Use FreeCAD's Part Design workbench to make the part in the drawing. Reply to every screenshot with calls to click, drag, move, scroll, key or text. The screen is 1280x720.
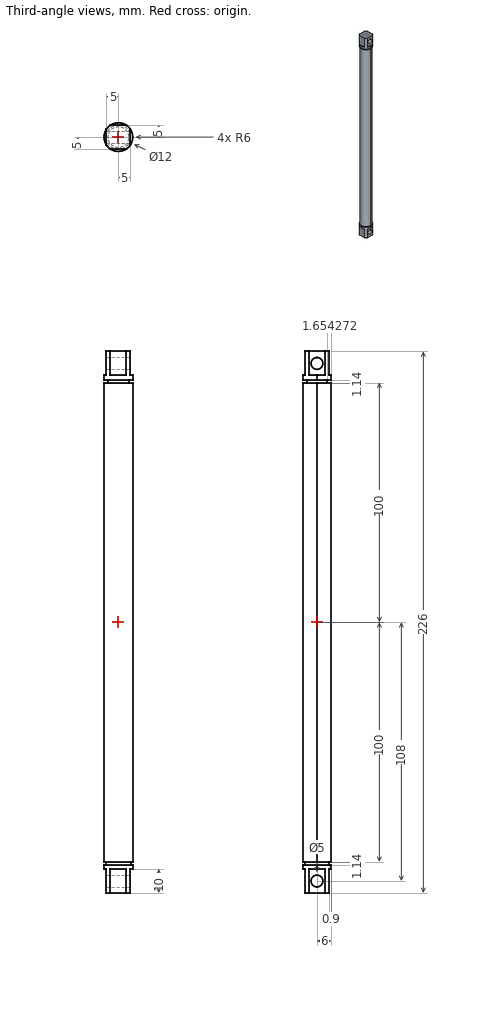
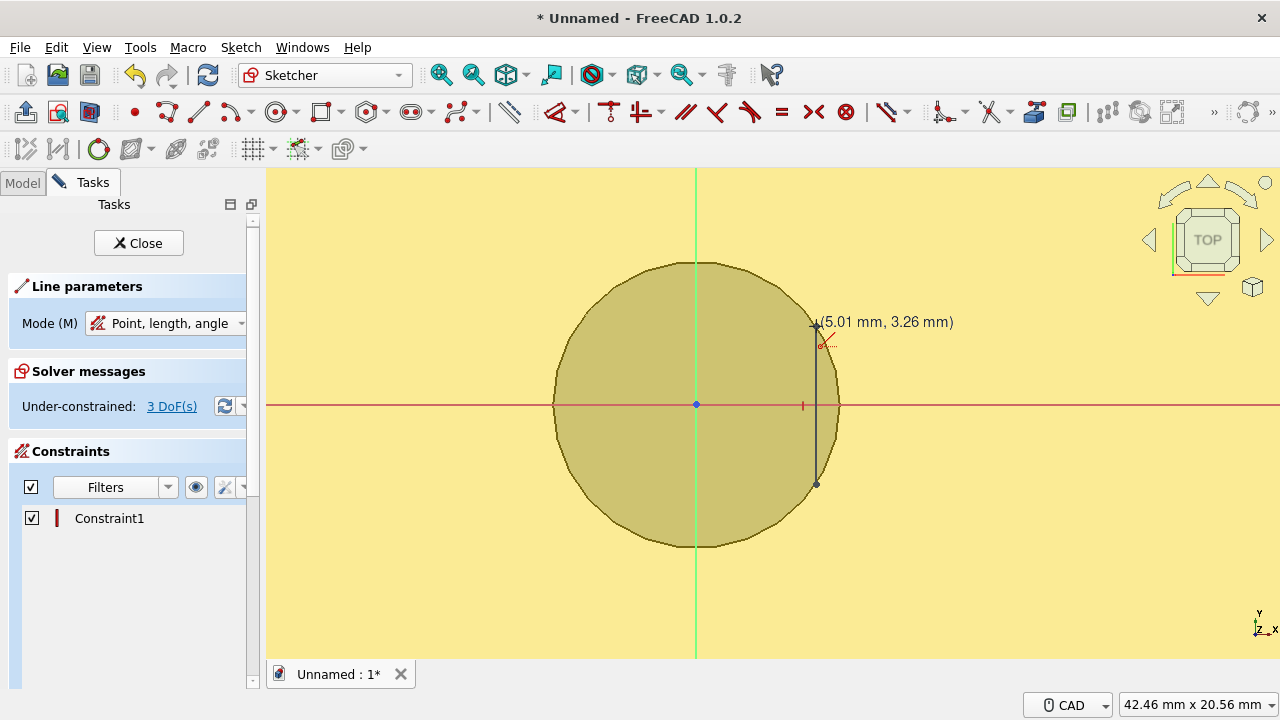
click(254, 112)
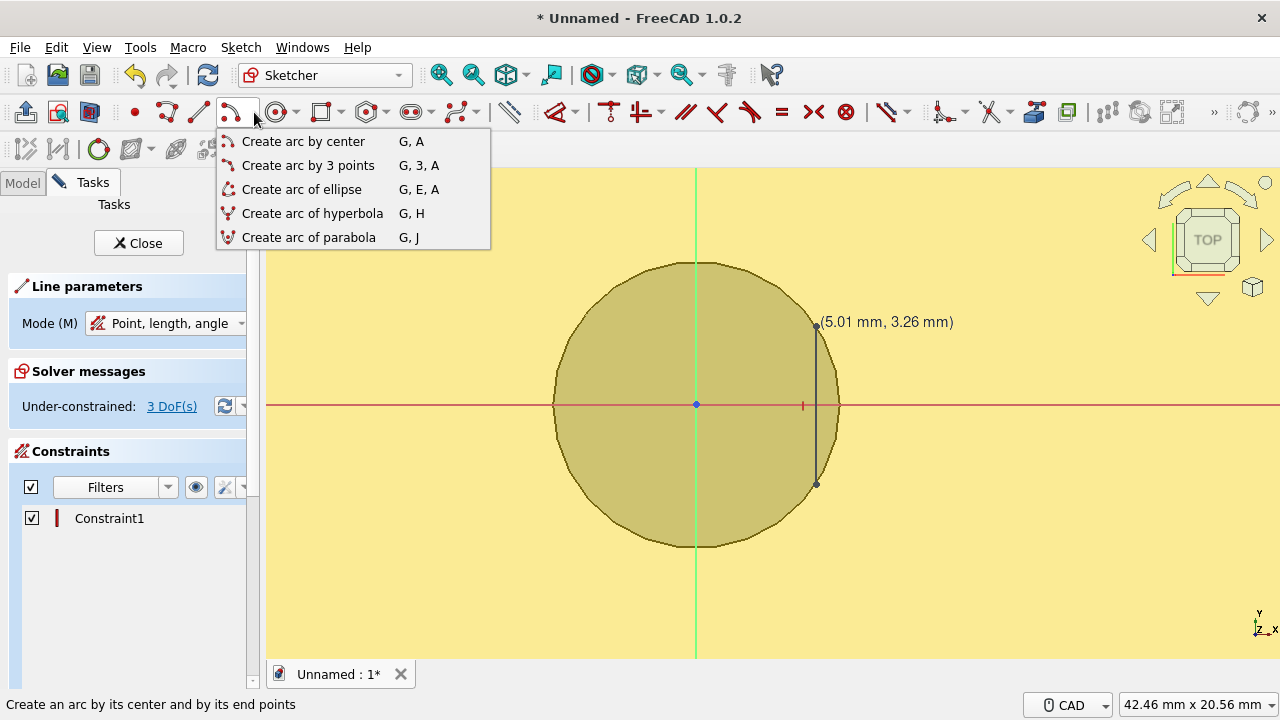
click(354, 165)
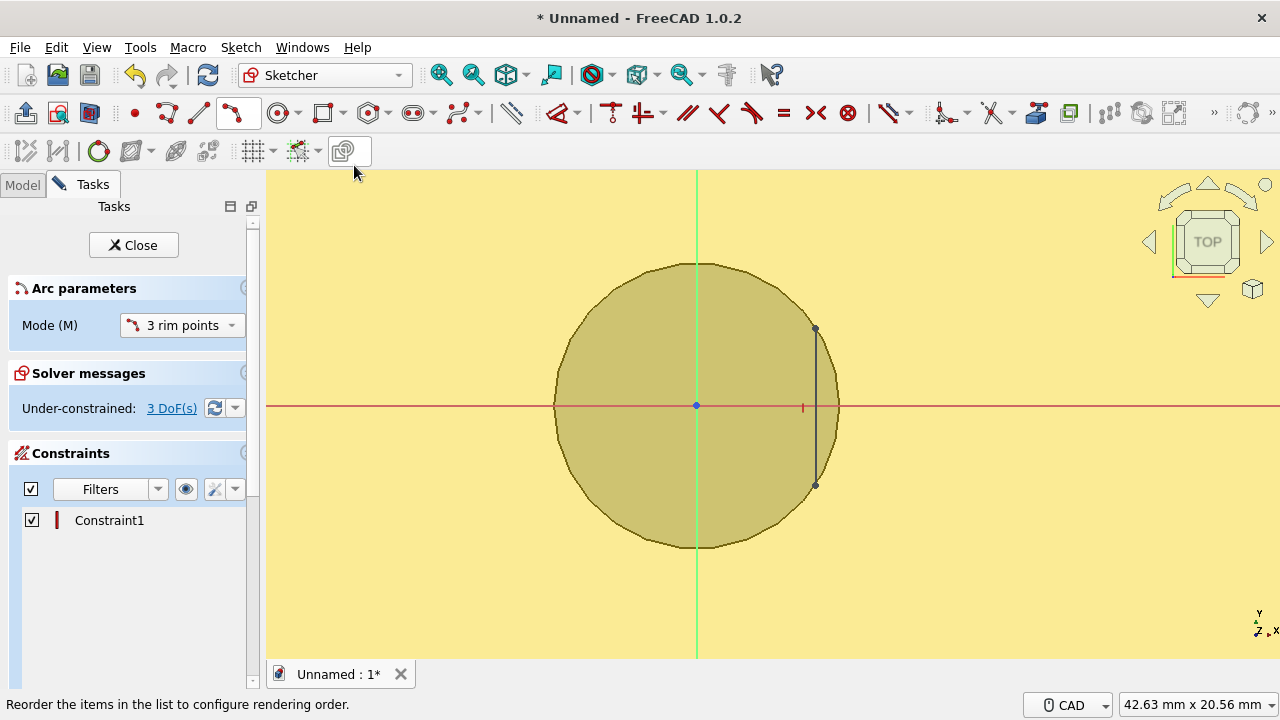
click(816, 328)
click(816, 486)
click(838, 423)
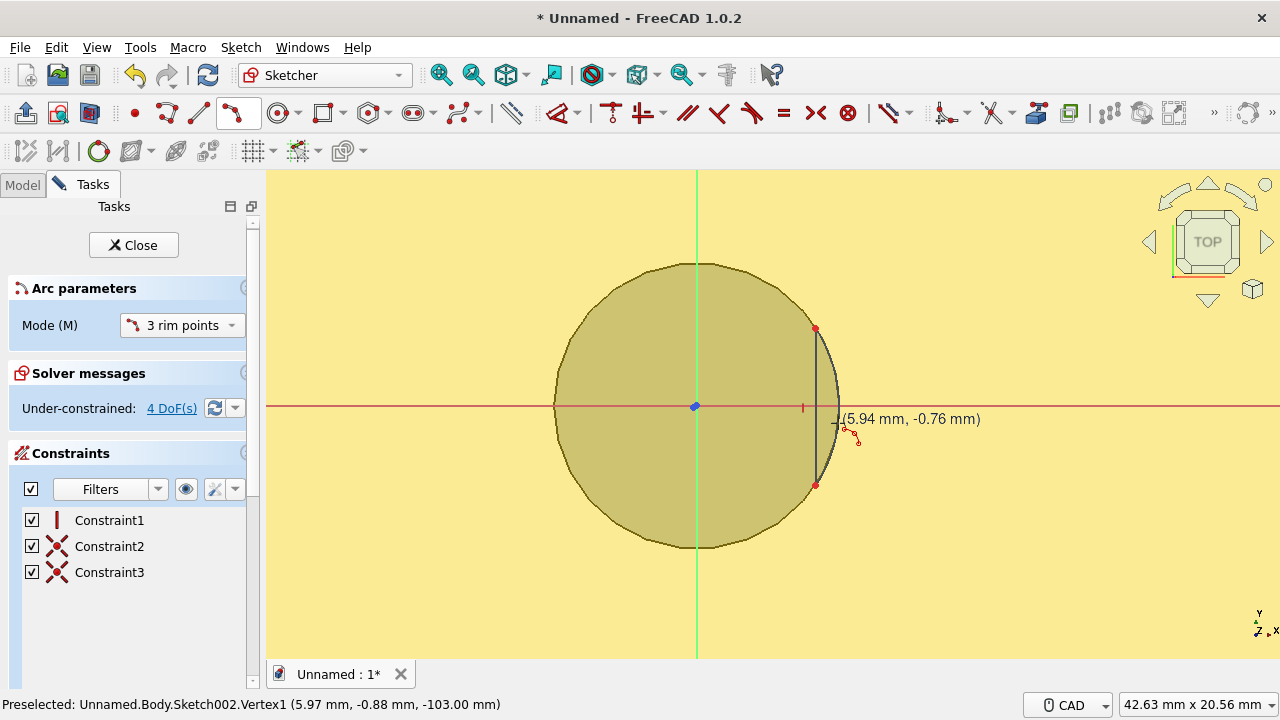
click(200, 114)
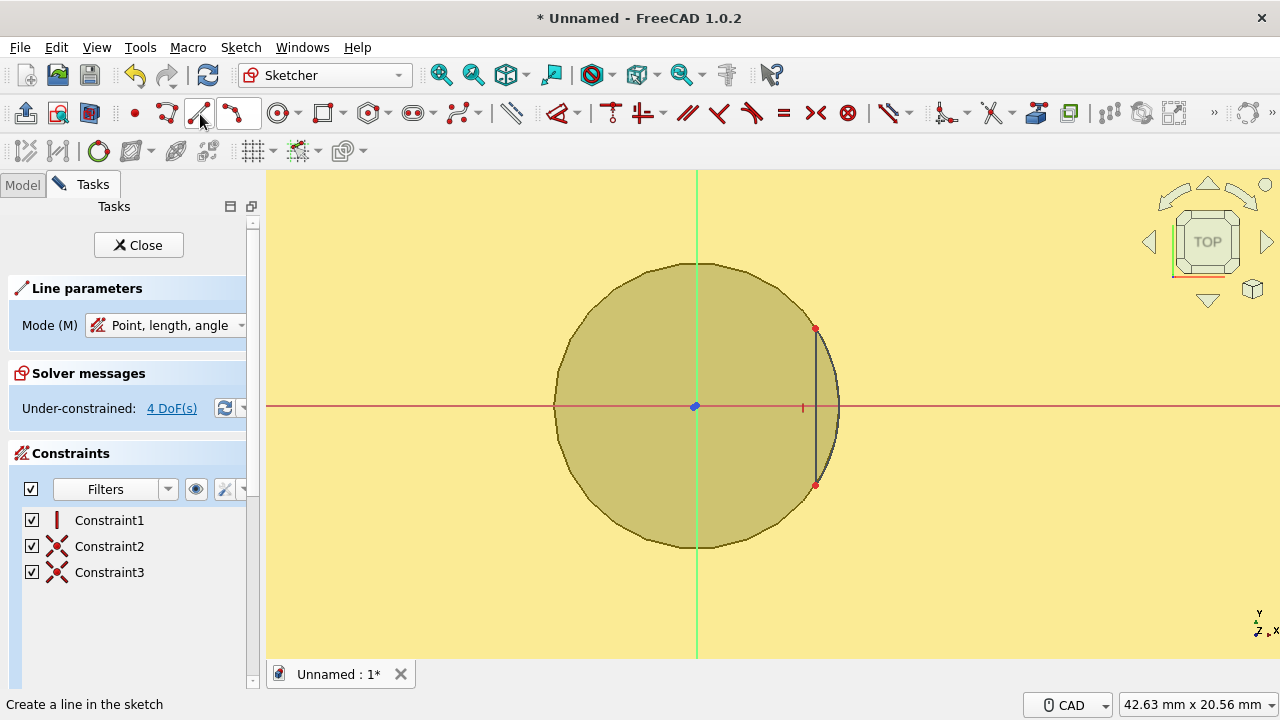
click(578, 327)
click(578, 485)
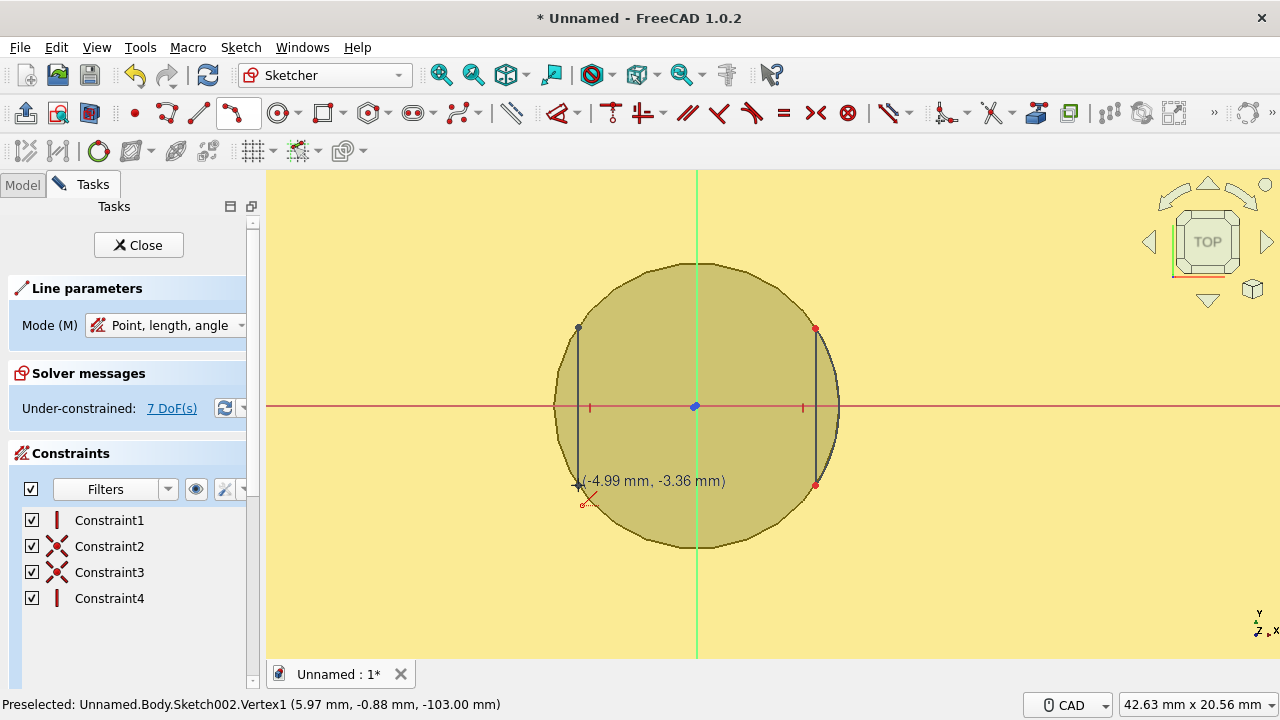
click(232, 114)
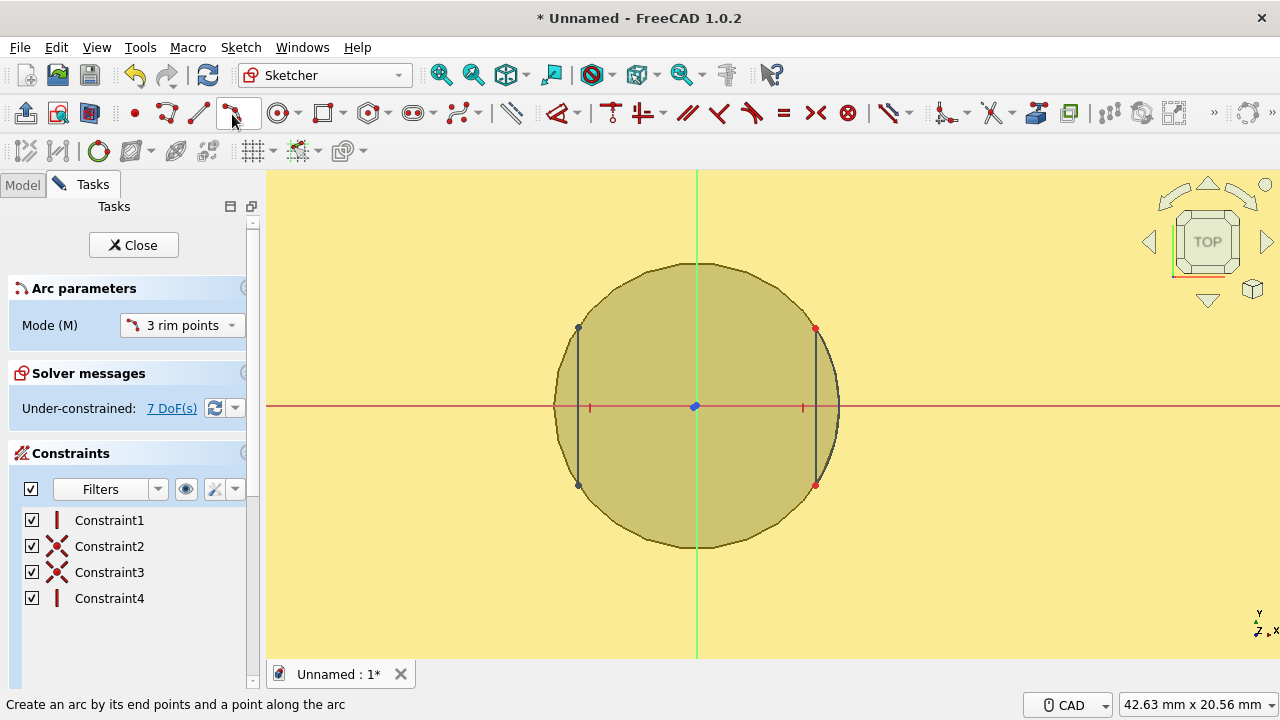
click(578, 486)
click(578, 328)
click(555, 389)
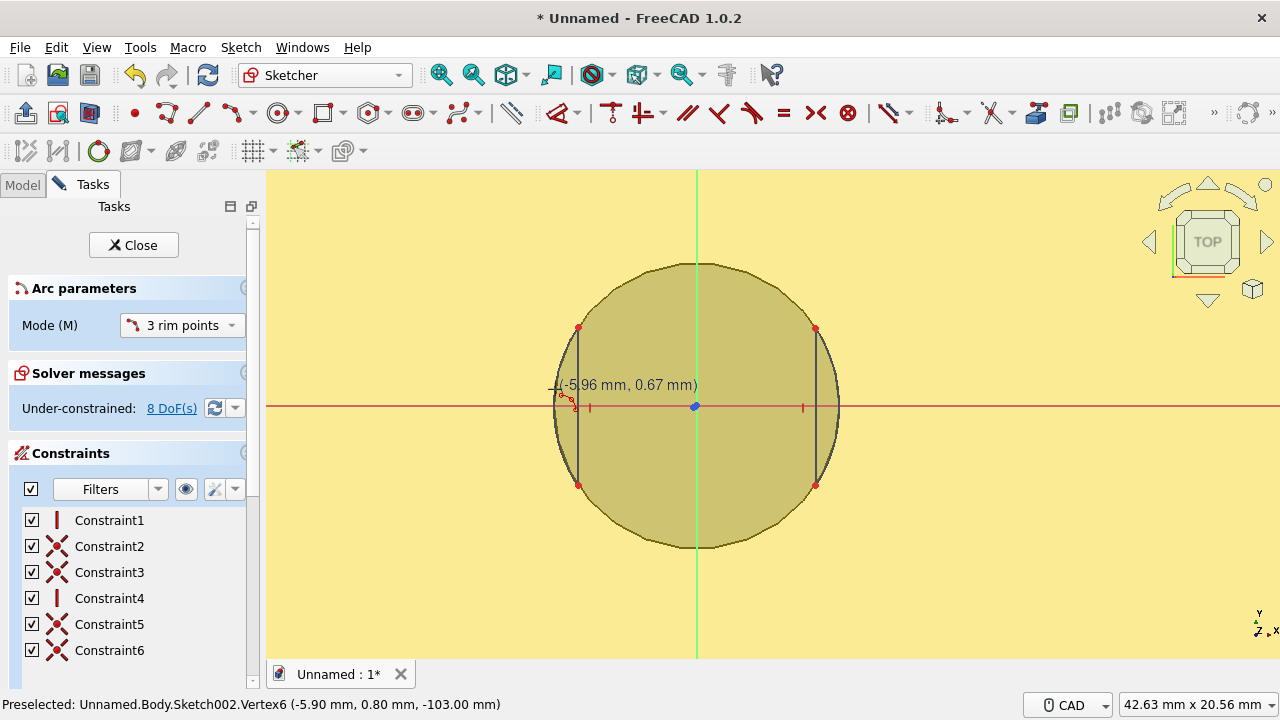
click(200, 114)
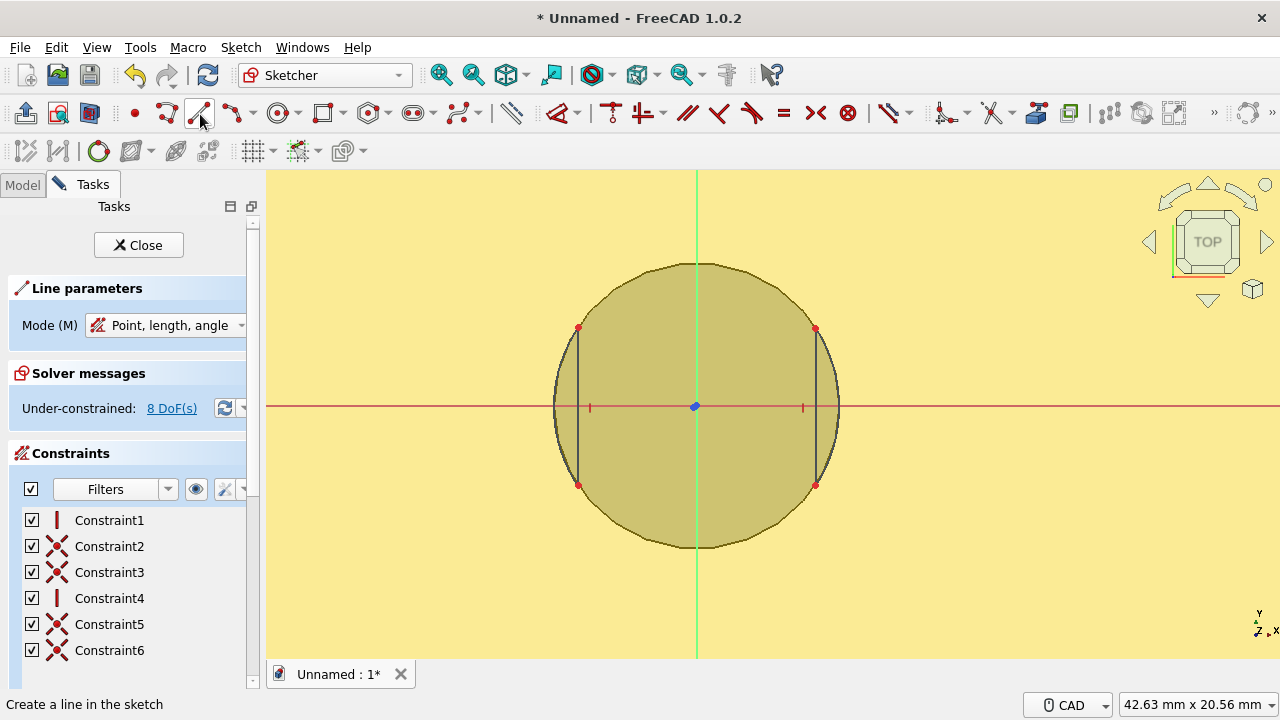
click(776, 287)
click(618, 287)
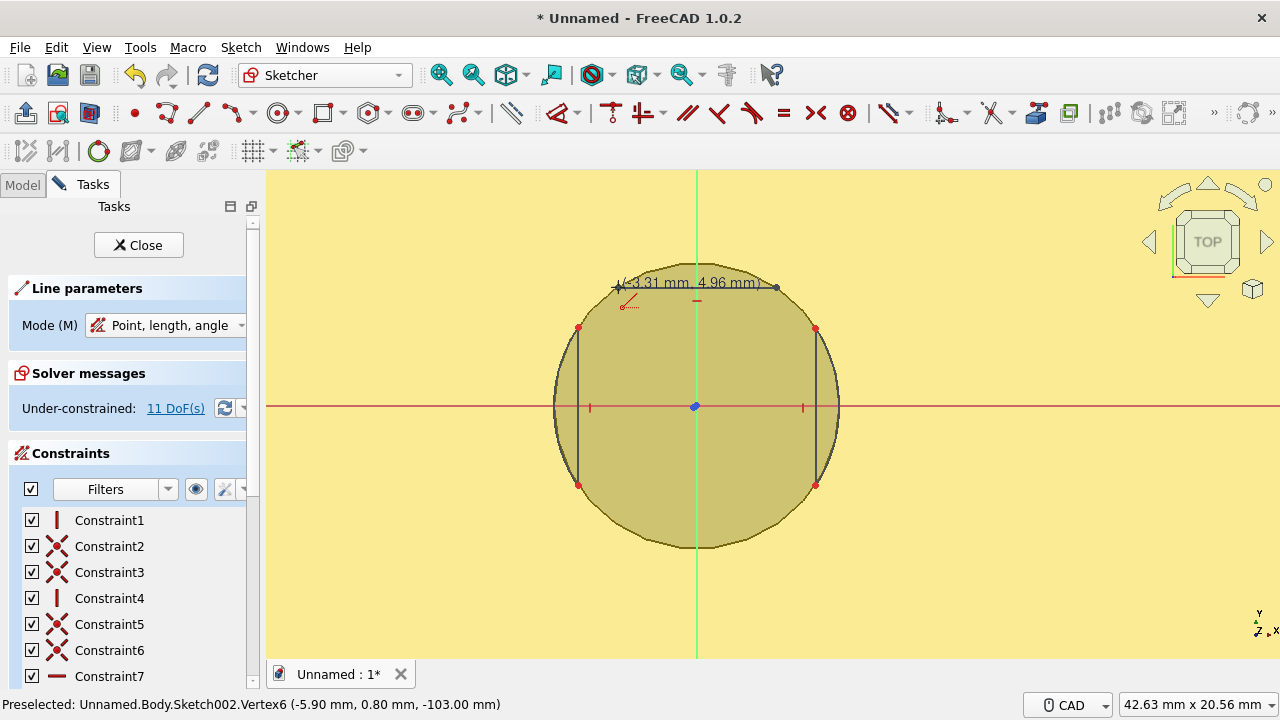
key(g)
key(3)
key(a)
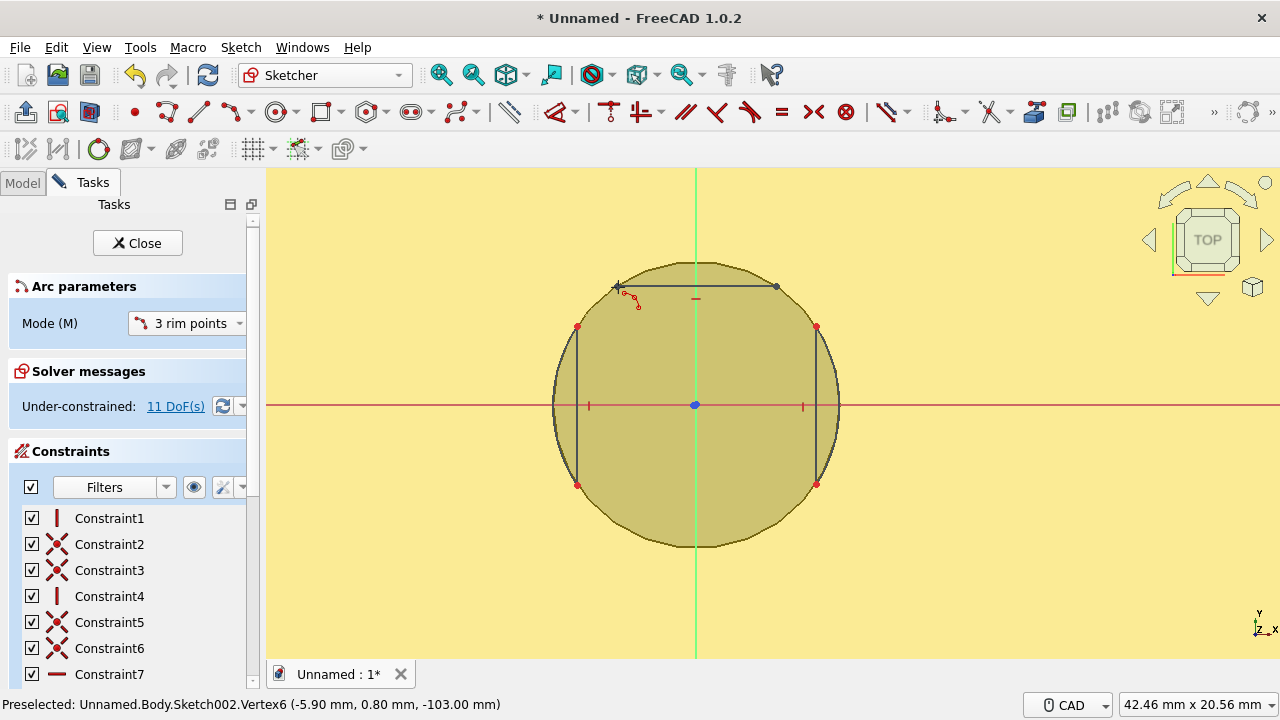
click(617, 286)
click(776, 286)
click(713, 263)